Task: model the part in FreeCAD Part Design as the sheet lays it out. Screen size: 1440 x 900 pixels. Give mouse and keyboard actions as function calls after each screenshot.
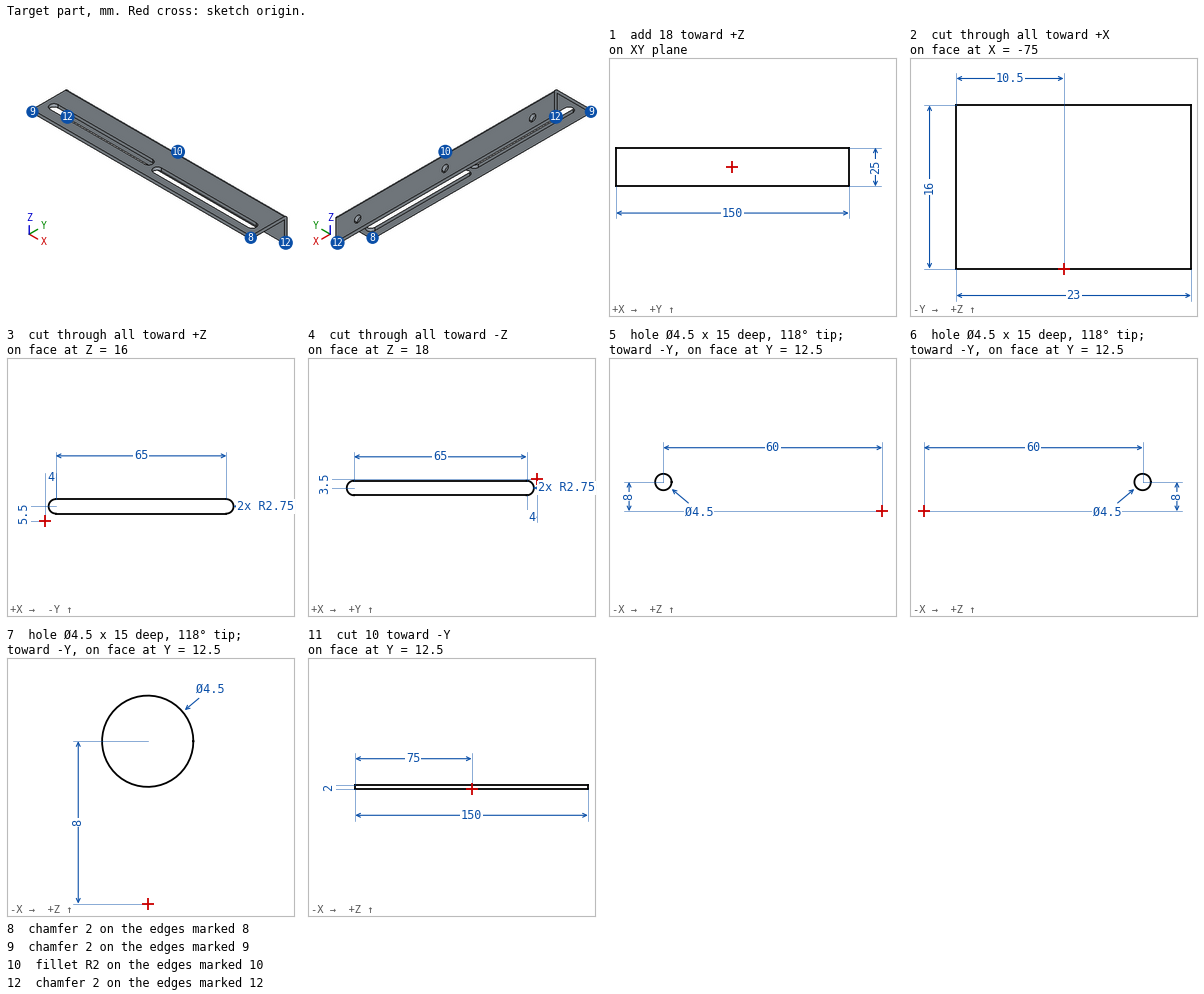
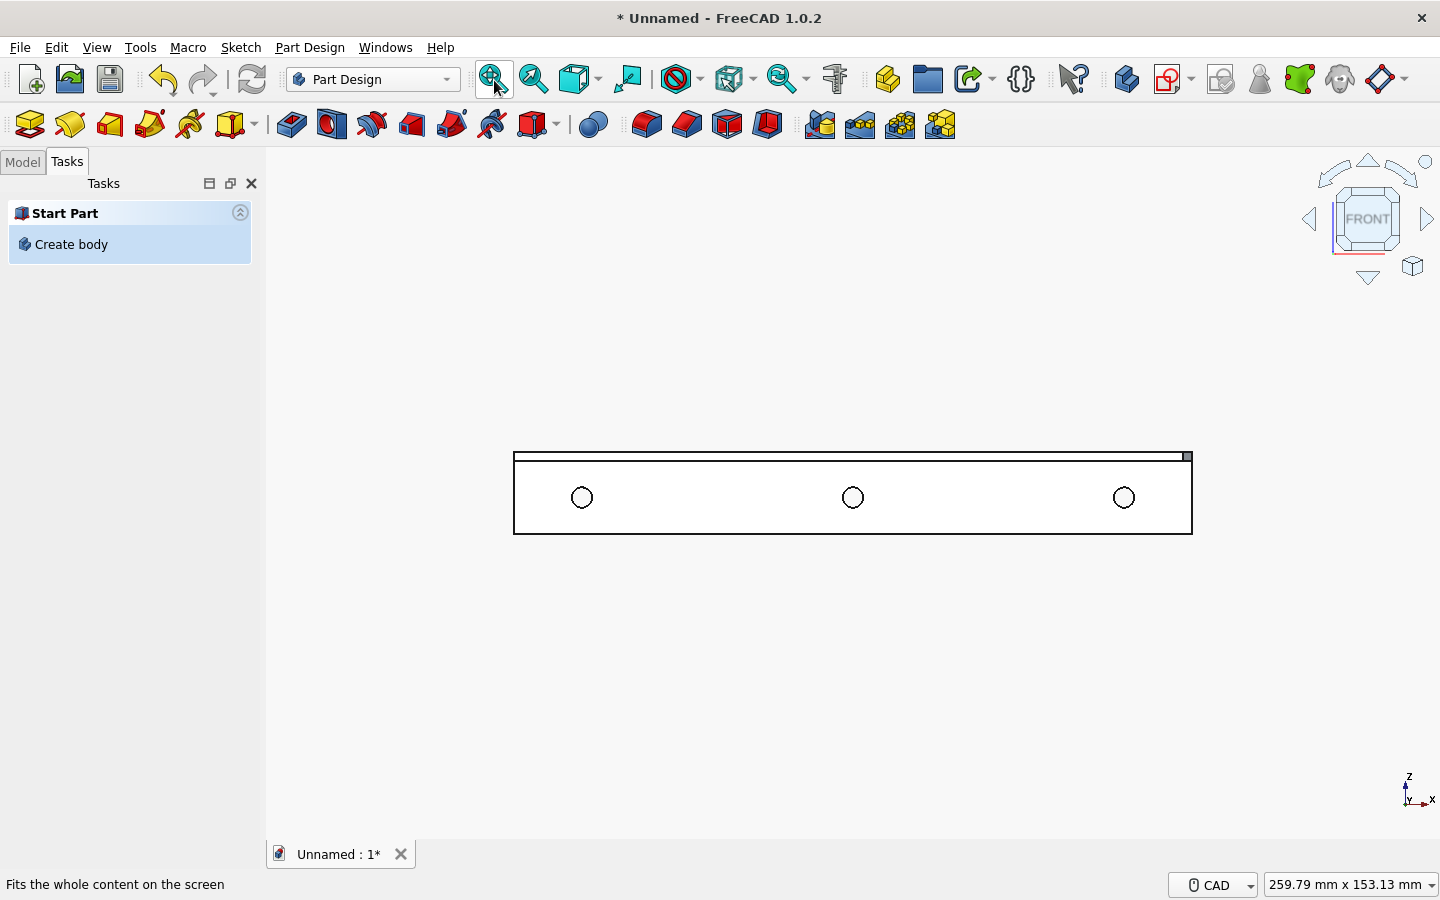
scroll(514, 456, up, 8)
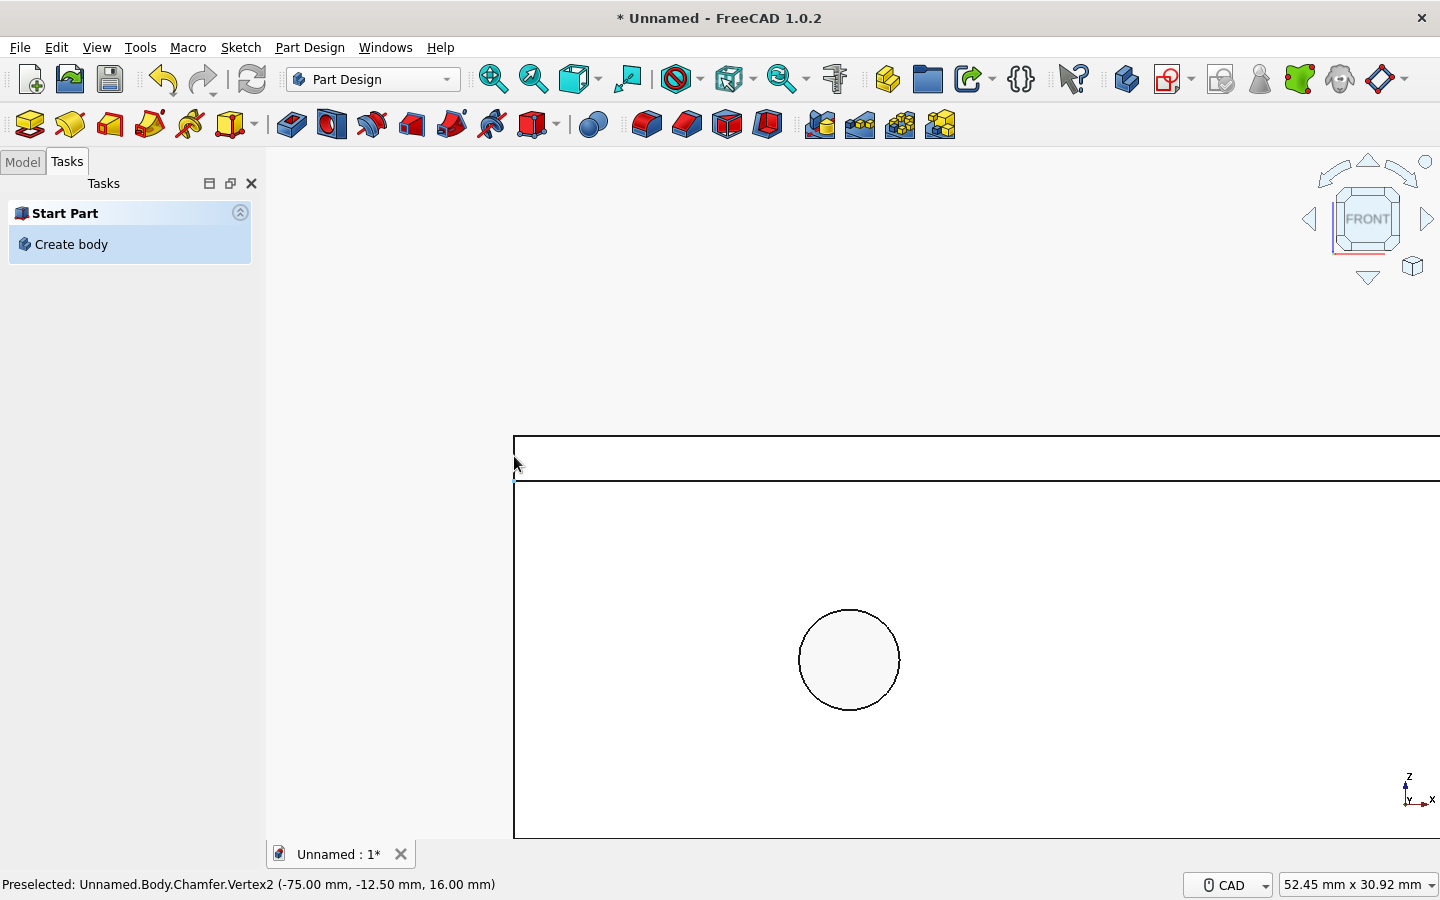
click(514, 457)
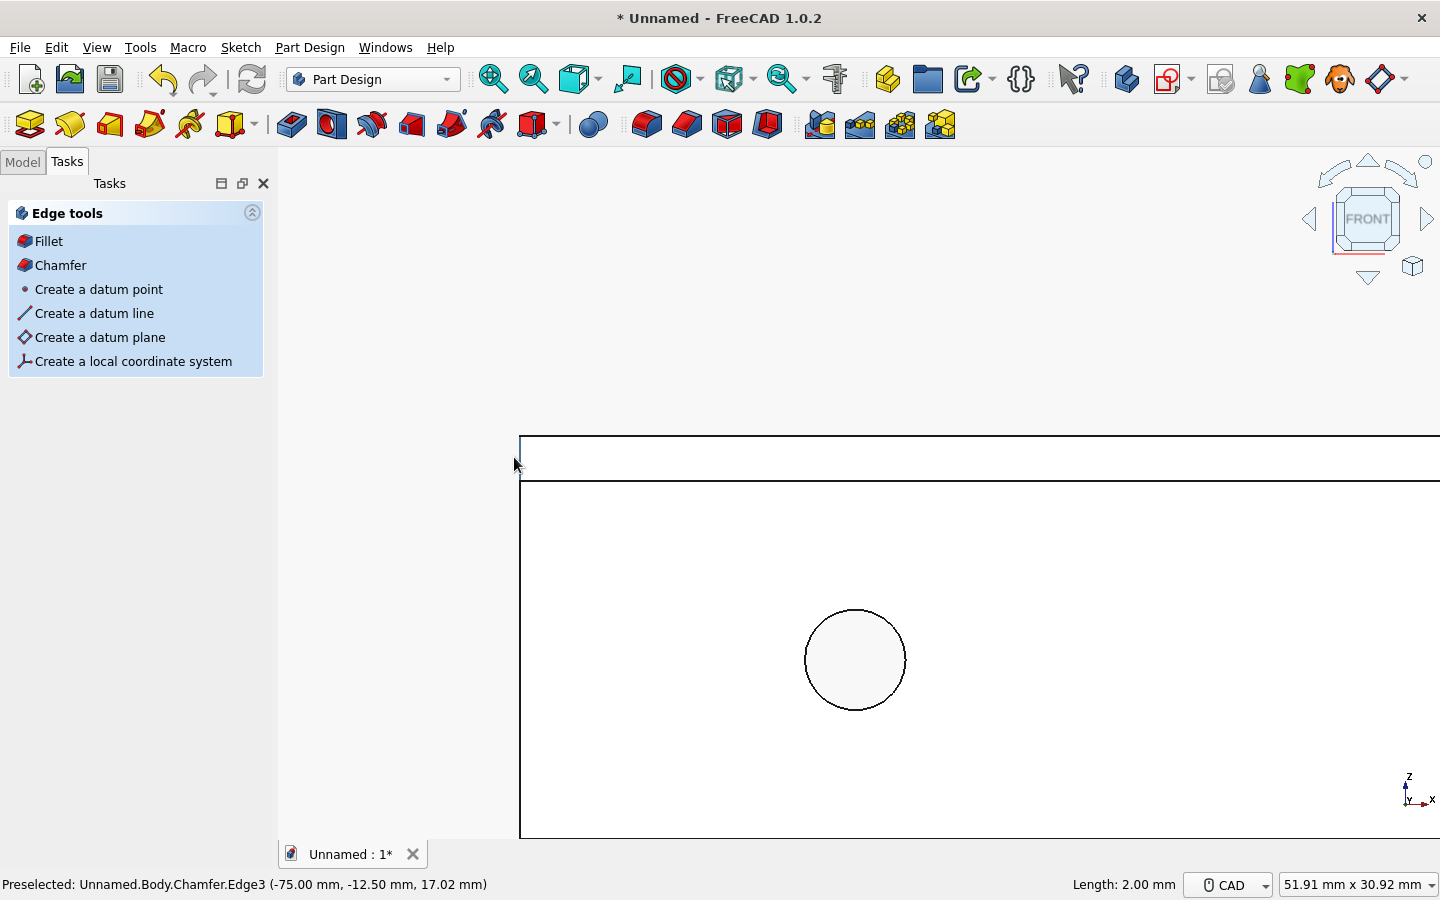
click(688, 124)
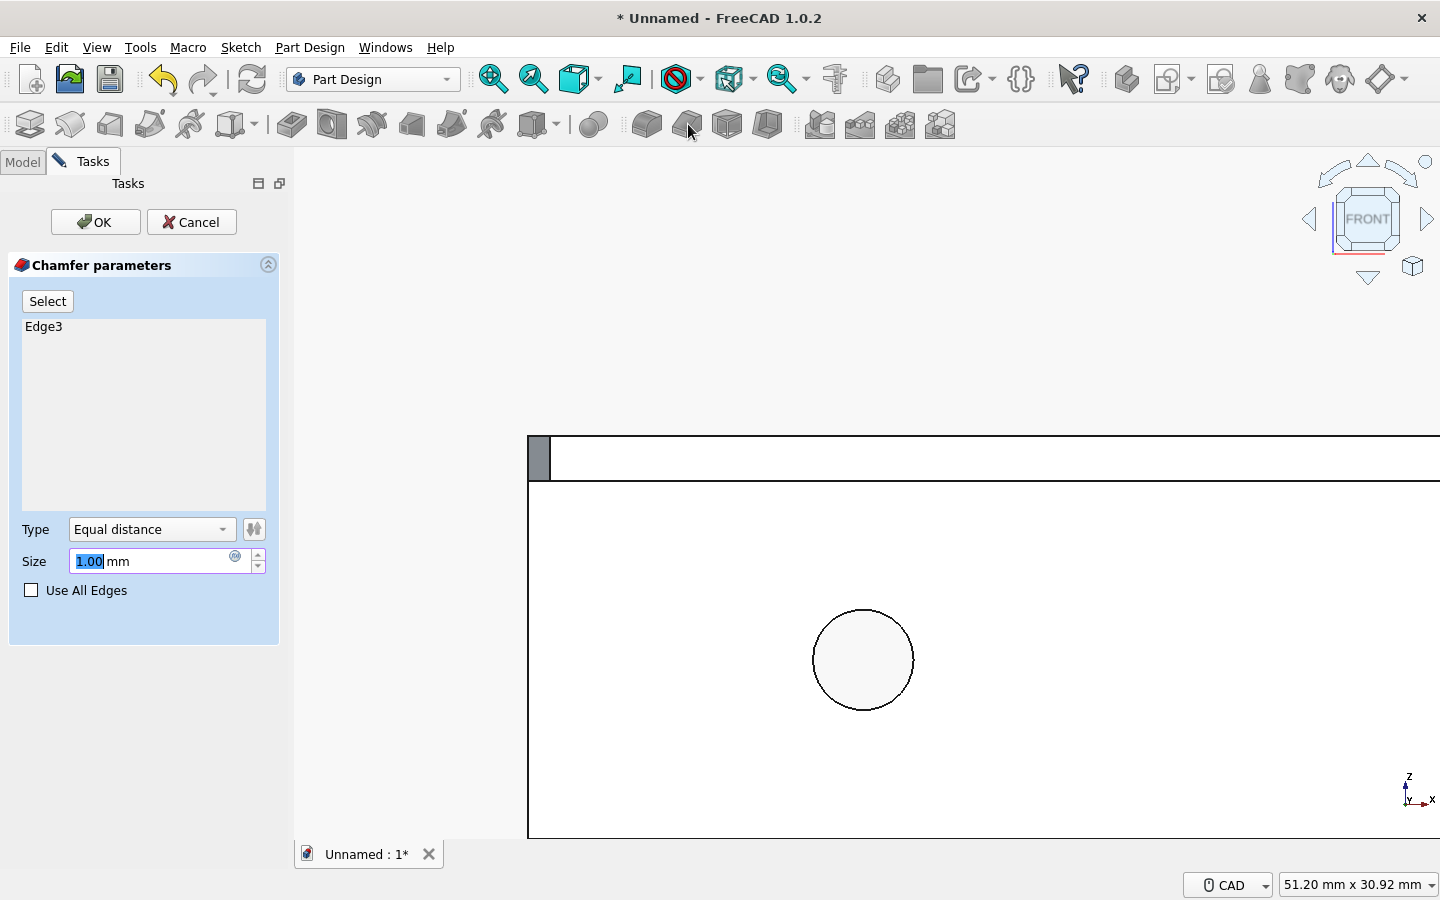
text(2)
key(Tab)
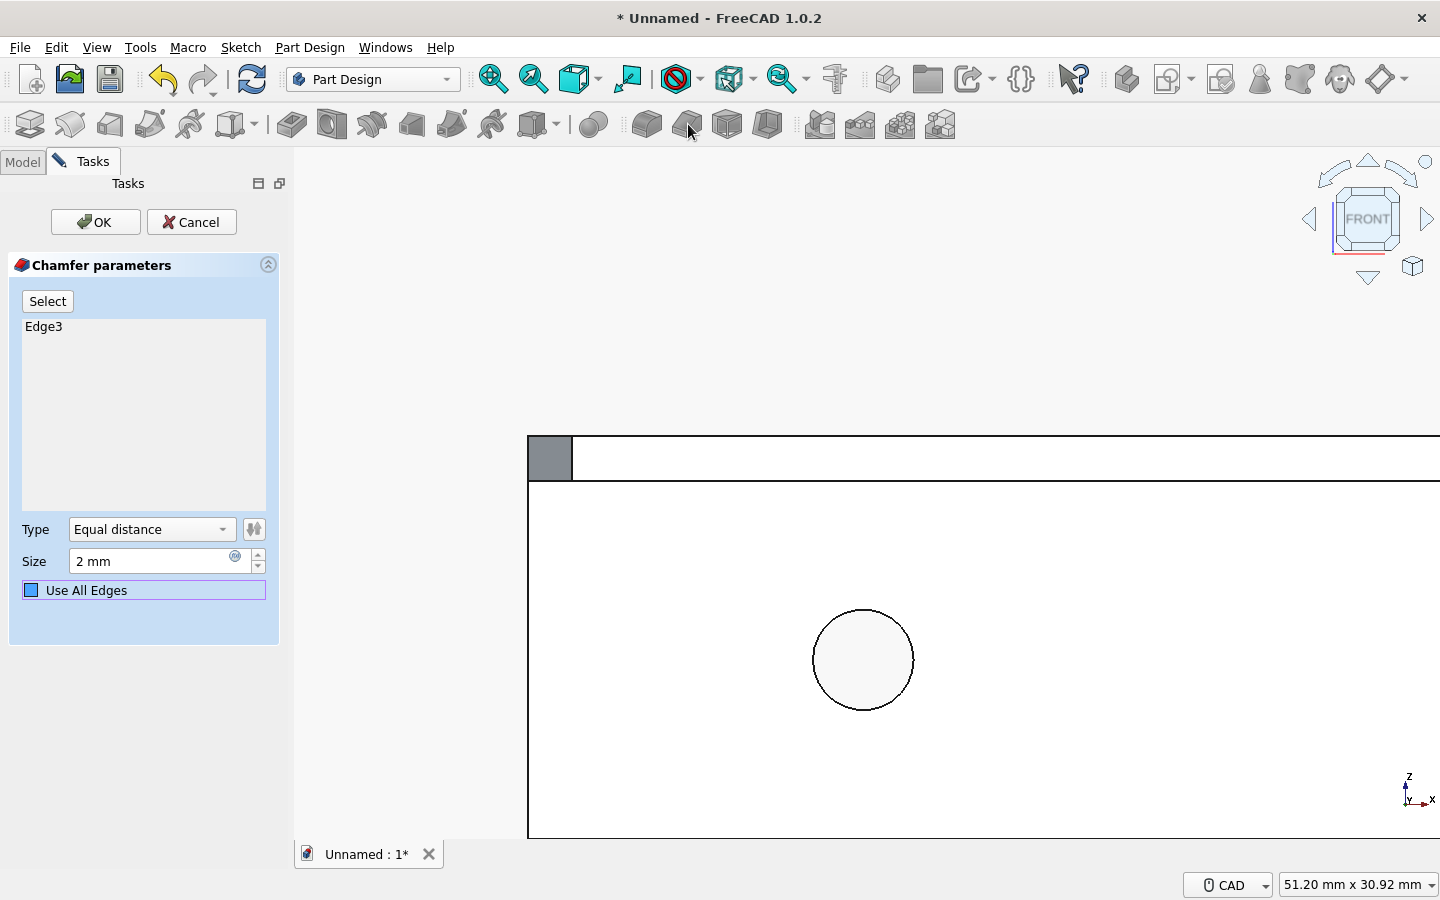
click(96, 222)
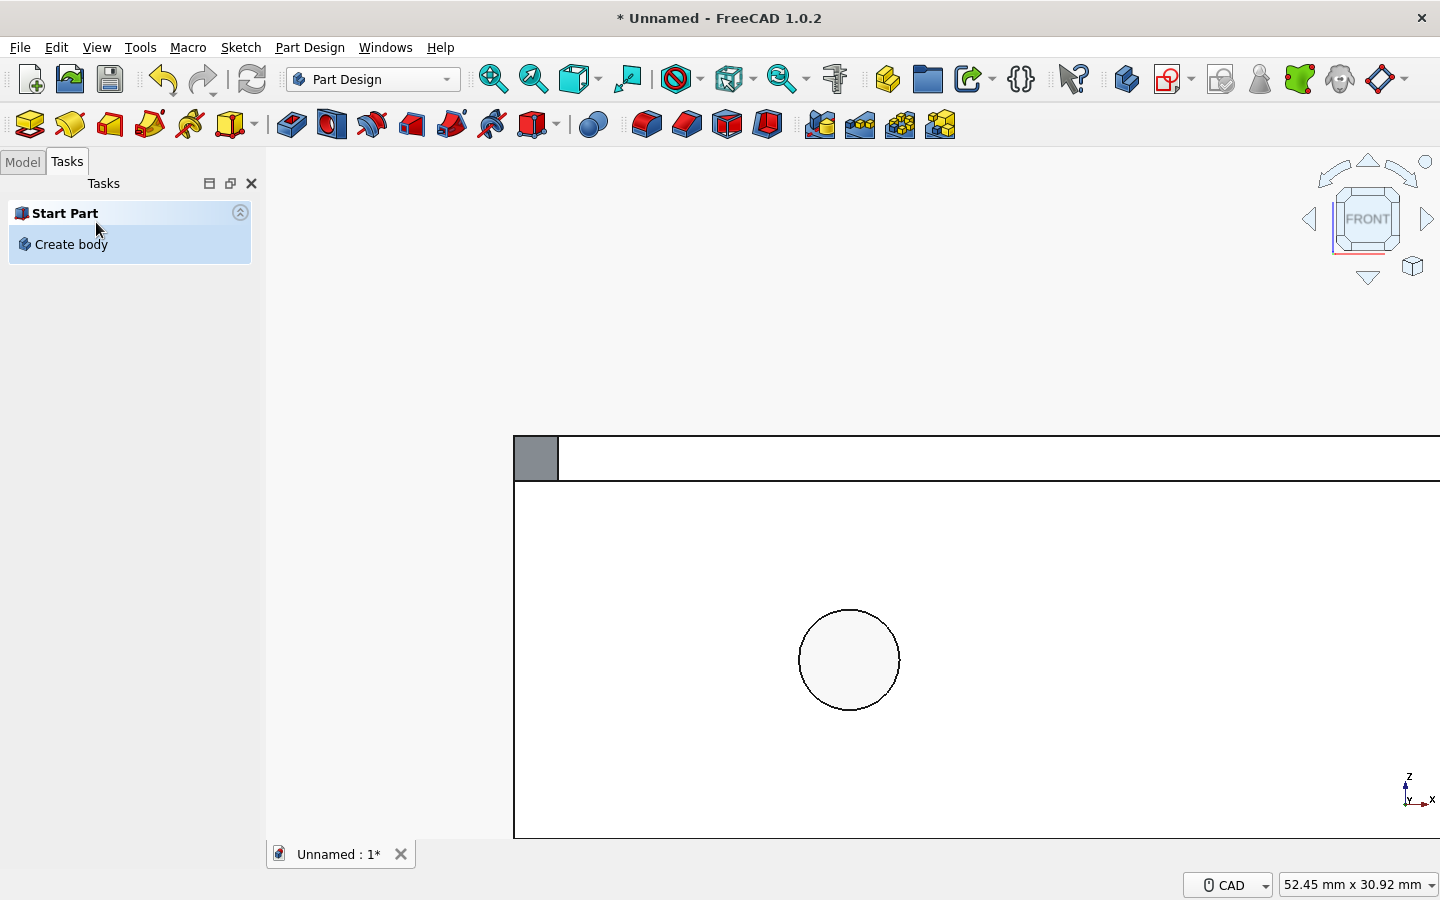
click(494, 80)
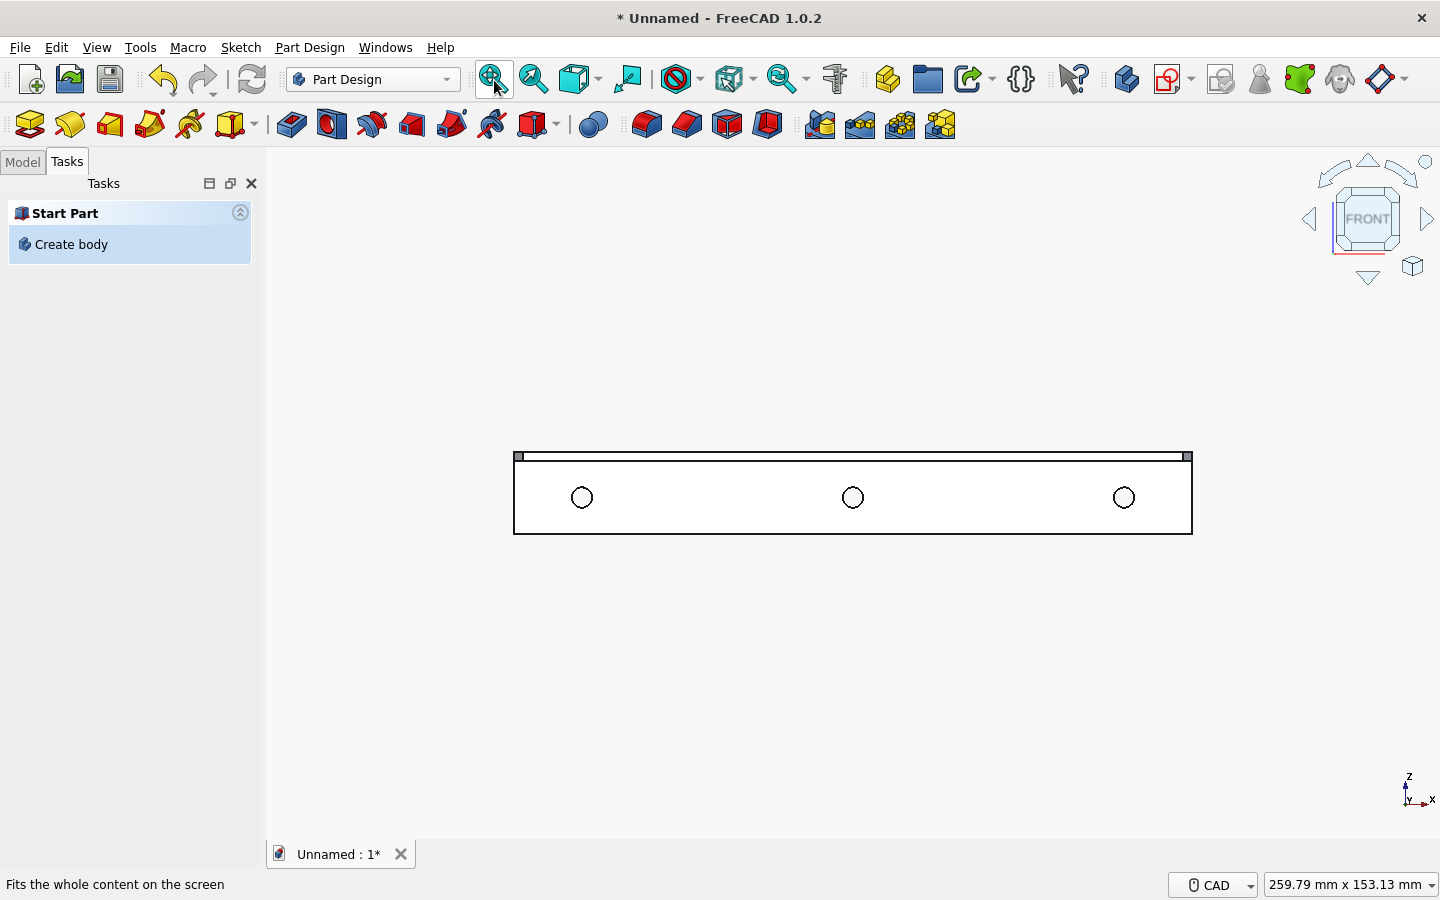
key(0)